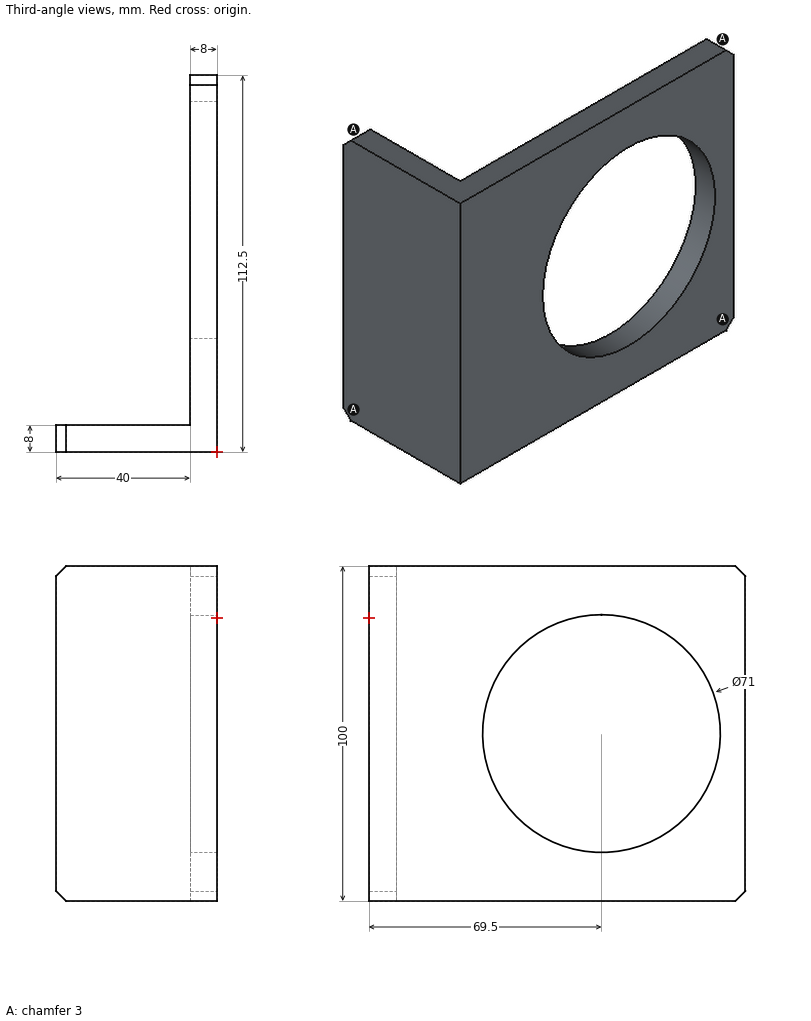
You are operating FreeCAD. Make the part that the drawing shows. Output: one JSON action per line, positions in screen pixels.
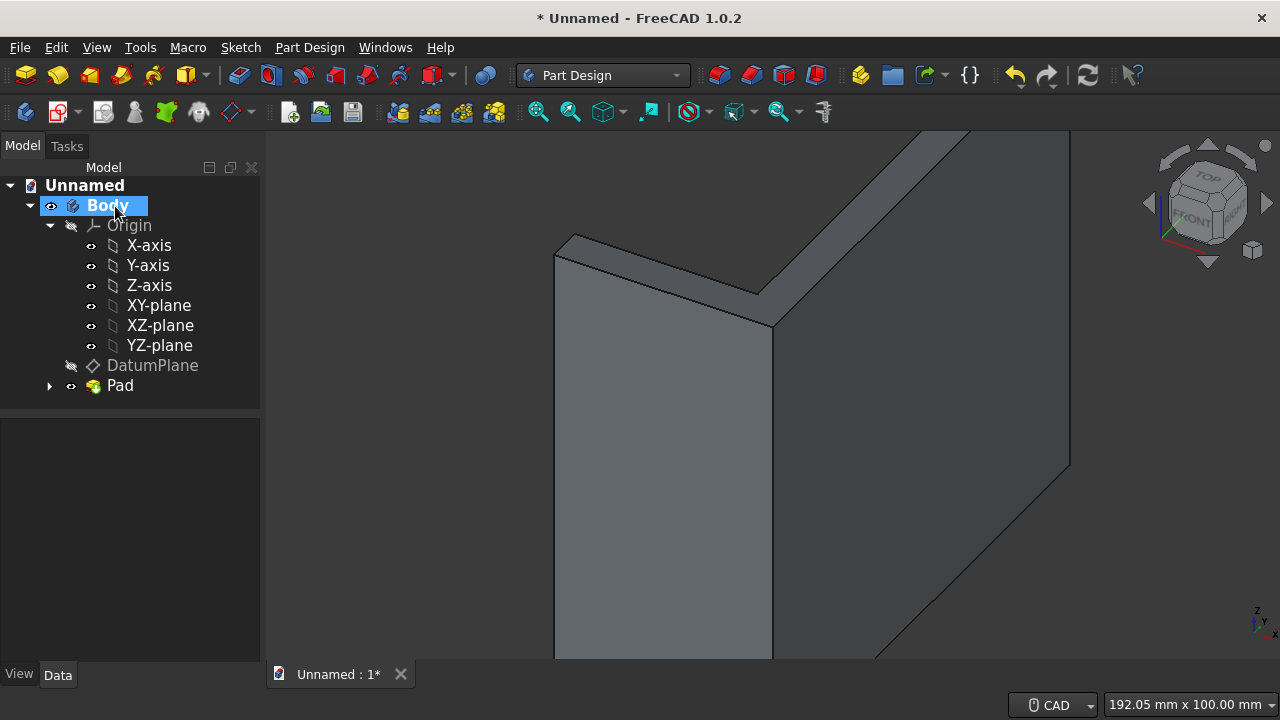
{"action": "left_click", "coordinate": [540, 112]}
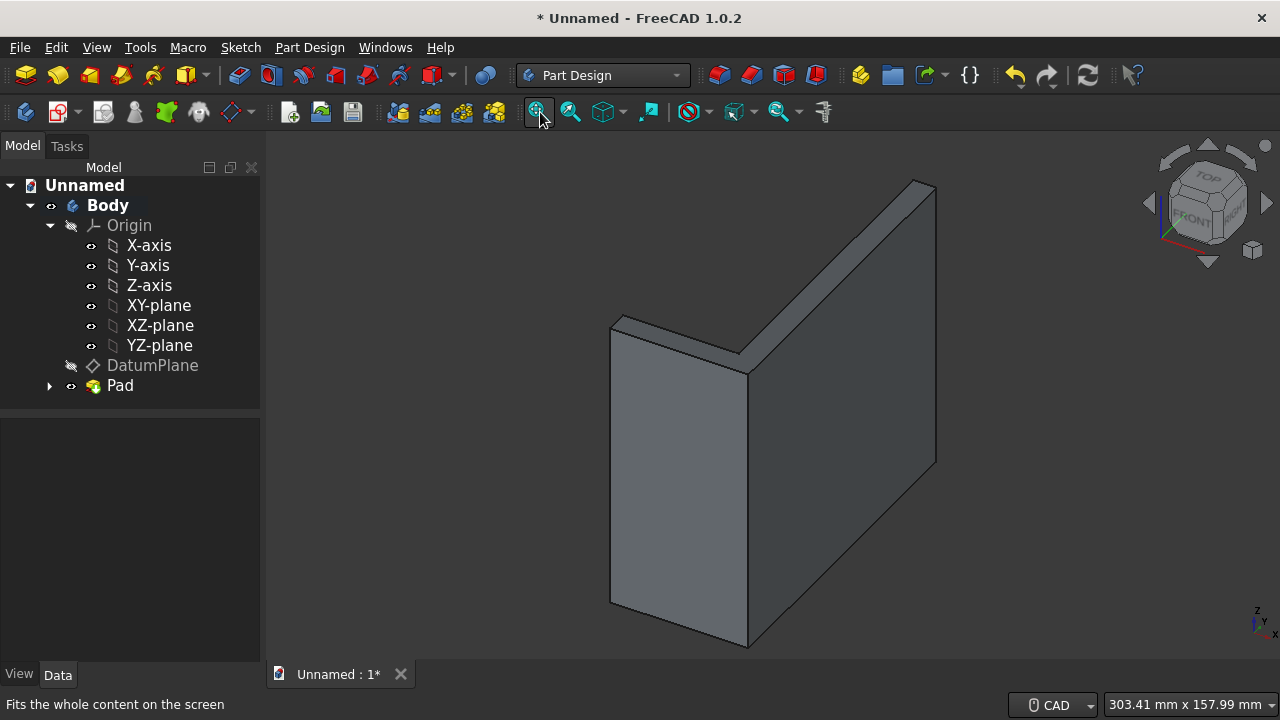
{"action": "key", "text": "0"}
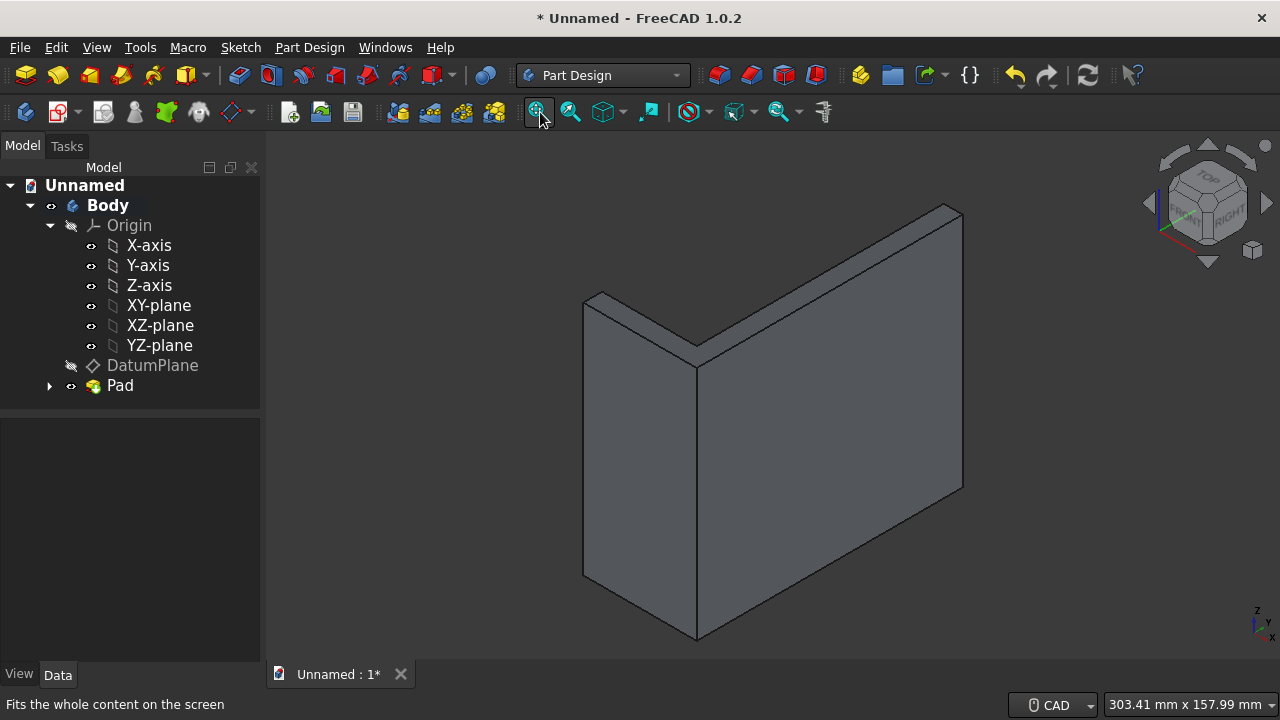
{"action": "key", "text": "2"}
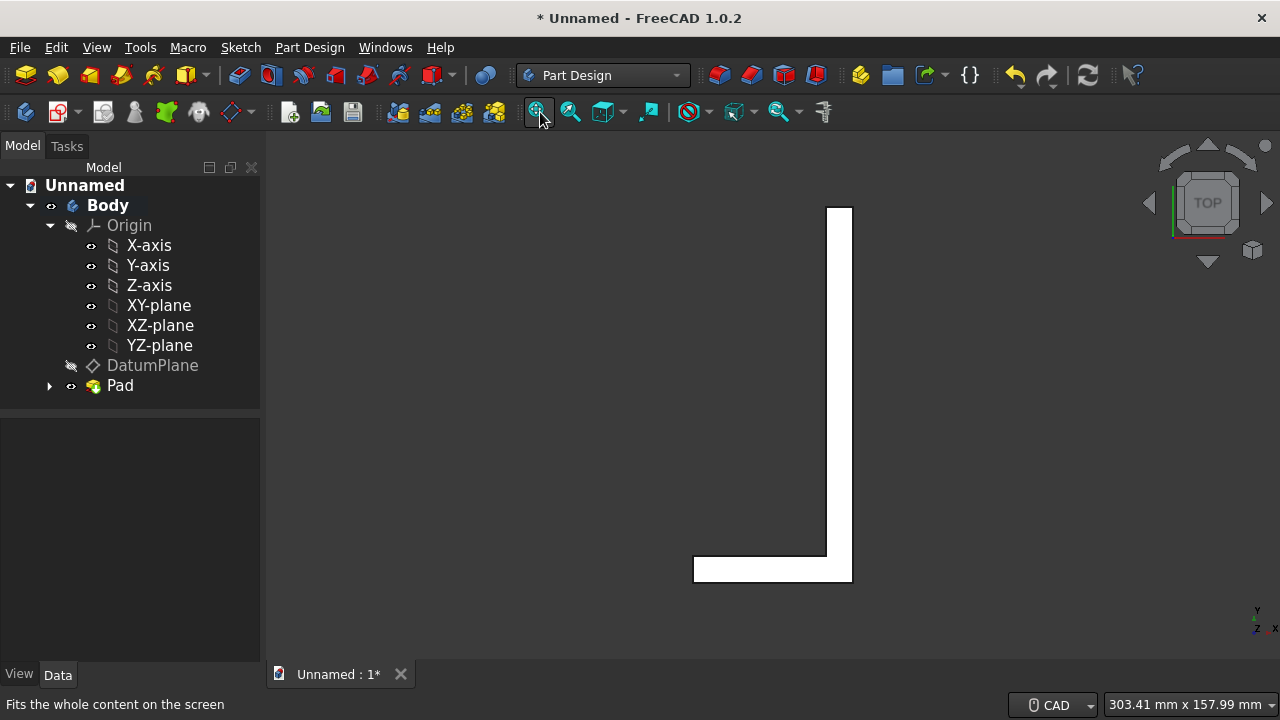
{"action": "left_click", "coordinate": [693, 569]}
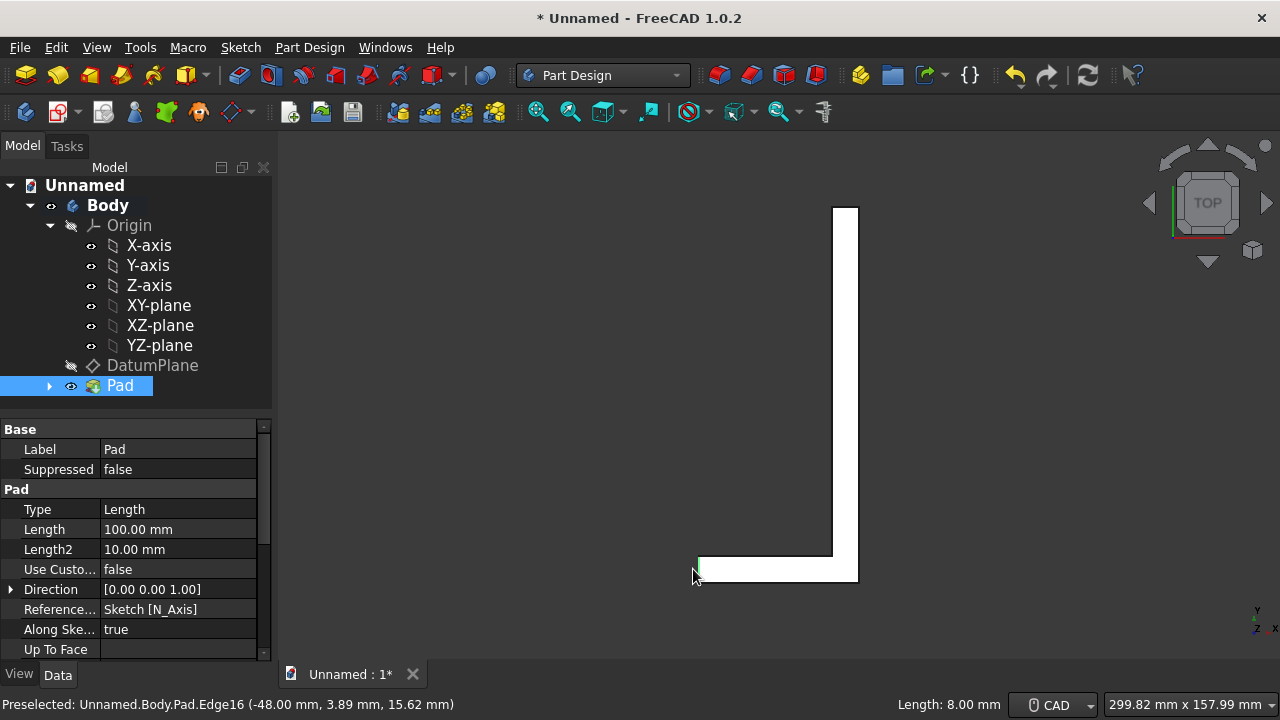
{"action": "left_click", "coordinate": [846, 206], "text": "ctrl"}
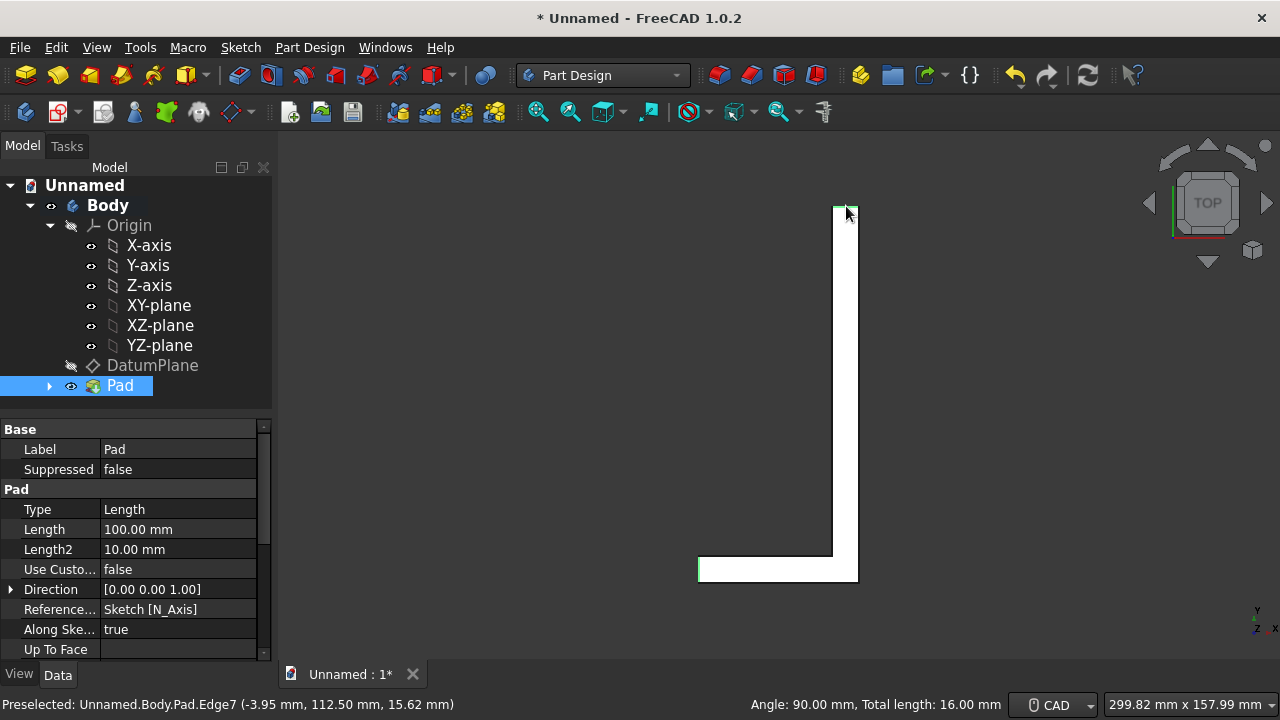
{"action": "key", "text": "1"}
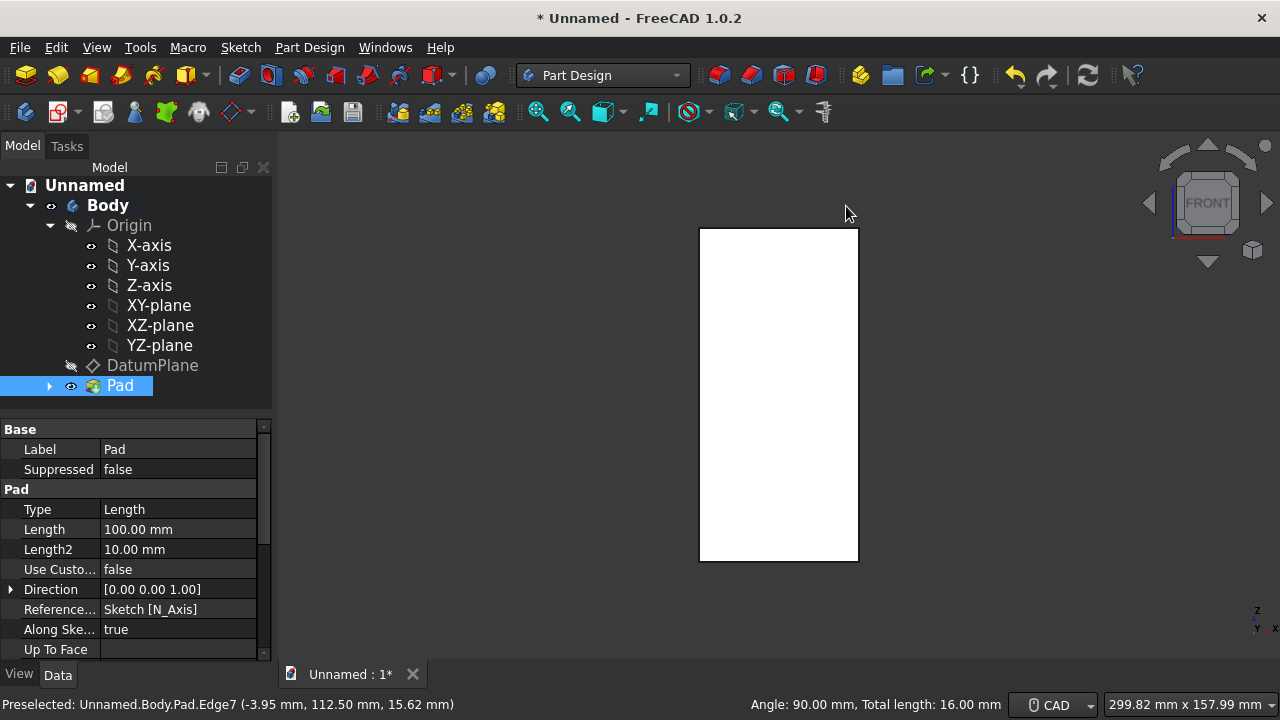
{"action": "key", "text": "3"}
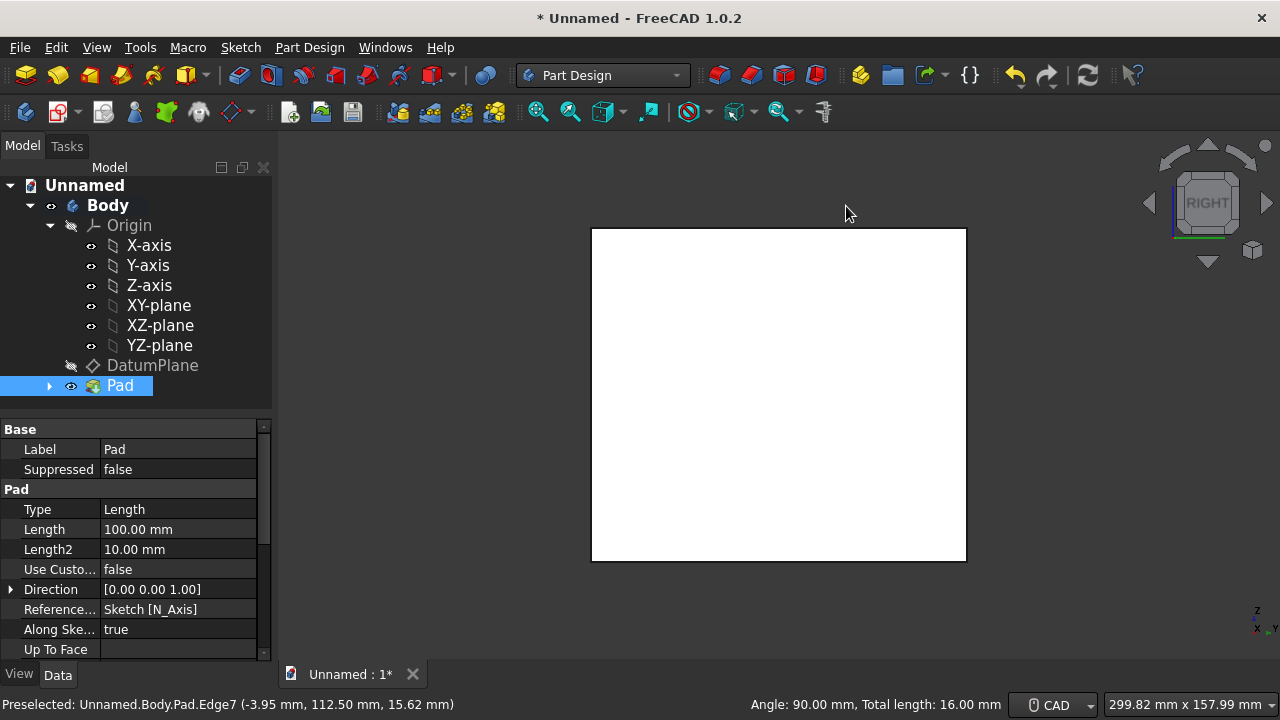
{"action": "key", "text": "5"}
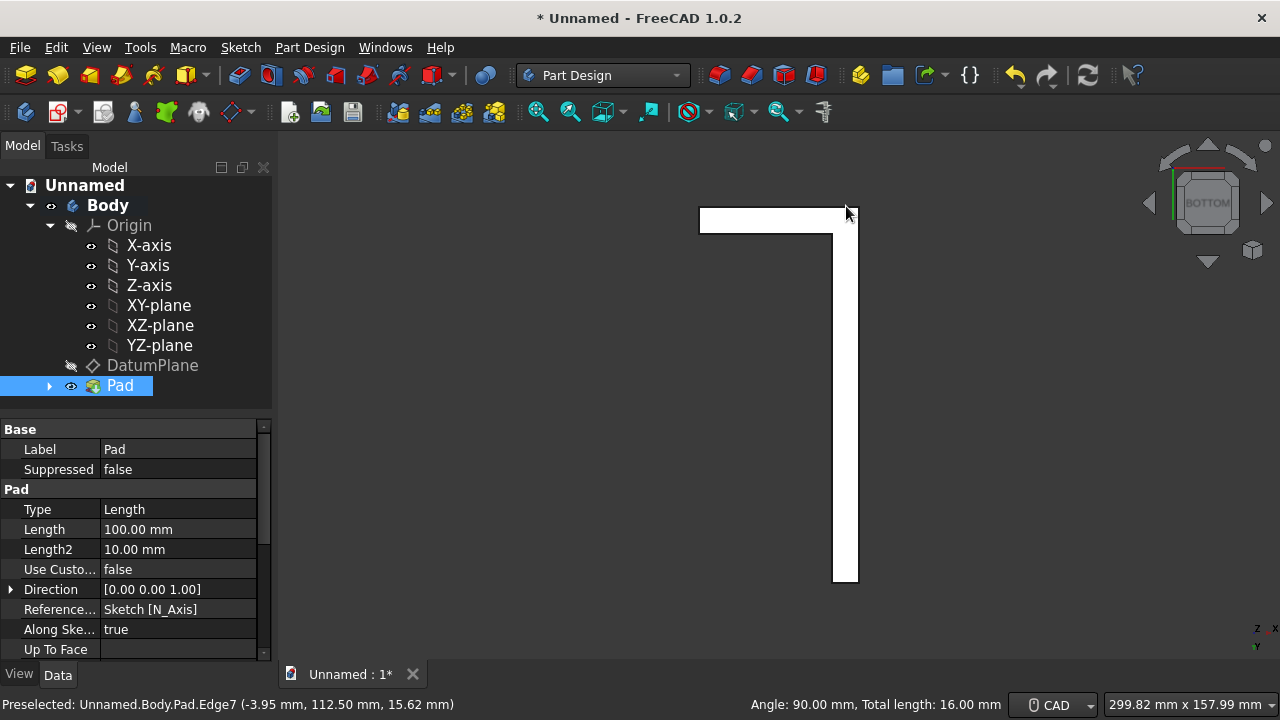
{"action": "left_click", "coordinate": [699, 219], "text": "ctrl"}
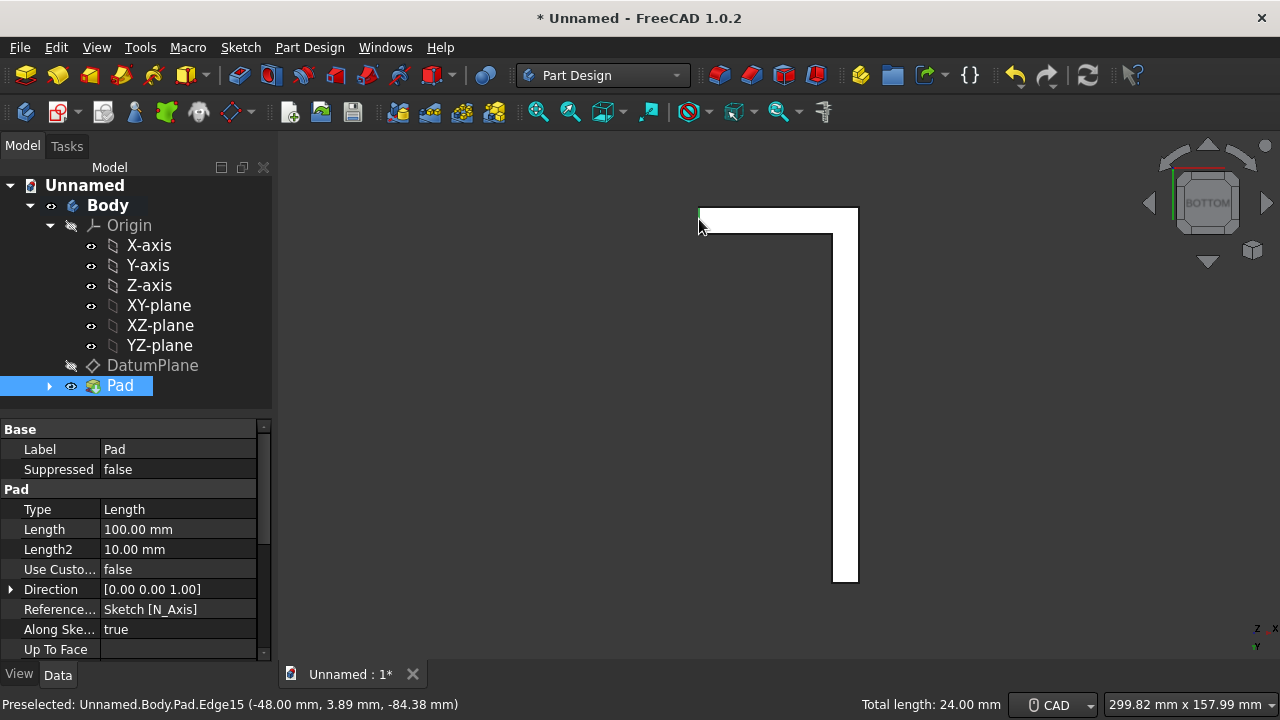
{"action": "left_click", "coordinate": [846, 582], "text": "ctrl"}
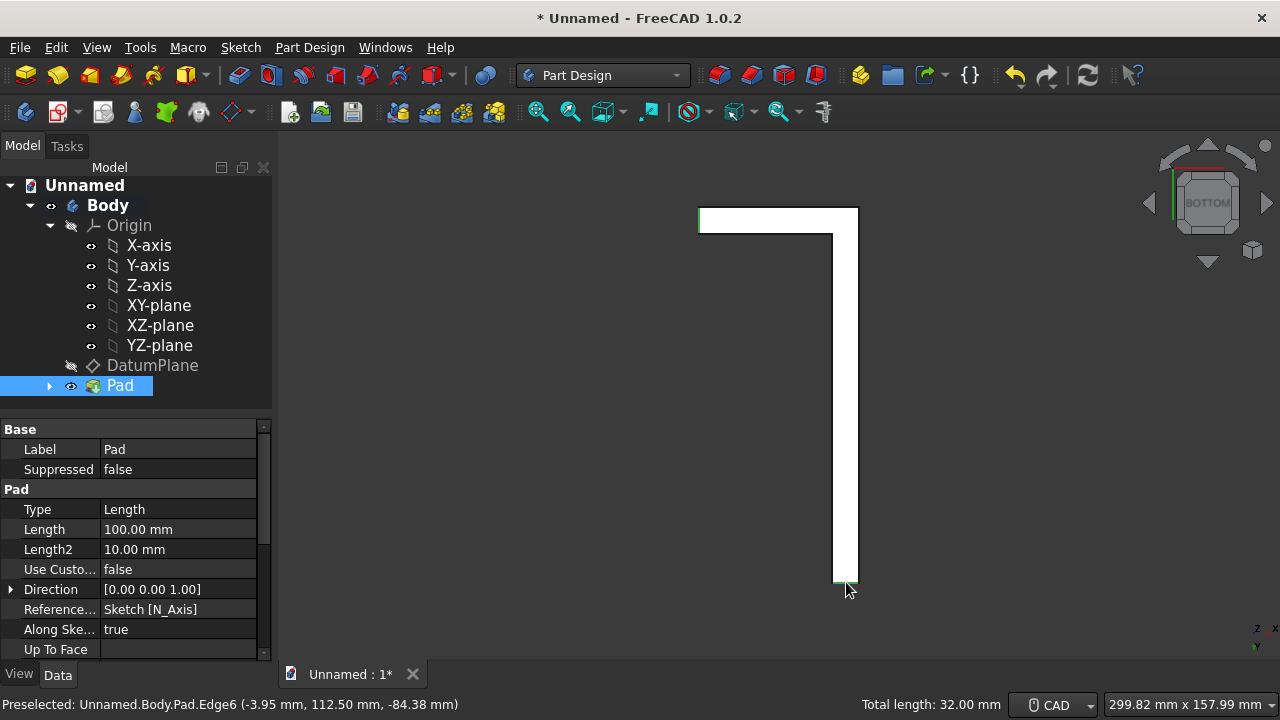
{"action": "left_click", "coordinate": [752, 76]}